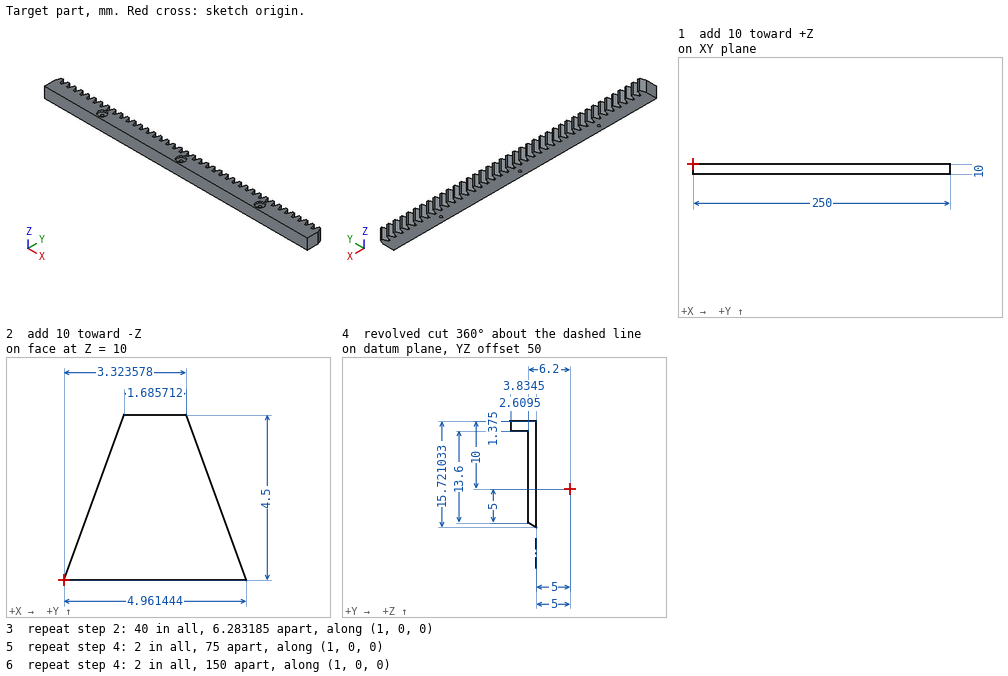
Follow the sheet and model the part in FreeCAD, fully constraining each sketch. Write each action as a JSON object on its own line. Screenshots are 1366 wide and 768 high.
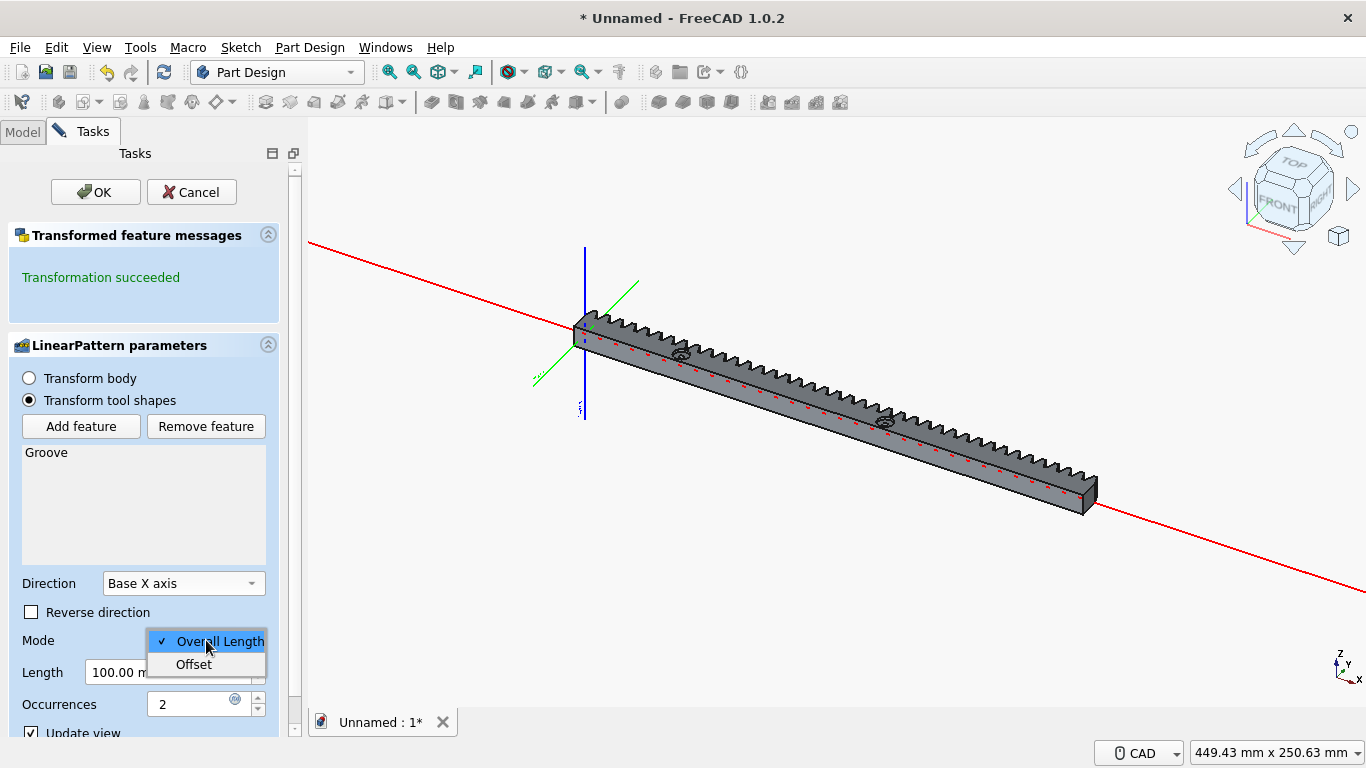
{"action": "left_click", "coordinate": [206, 664]}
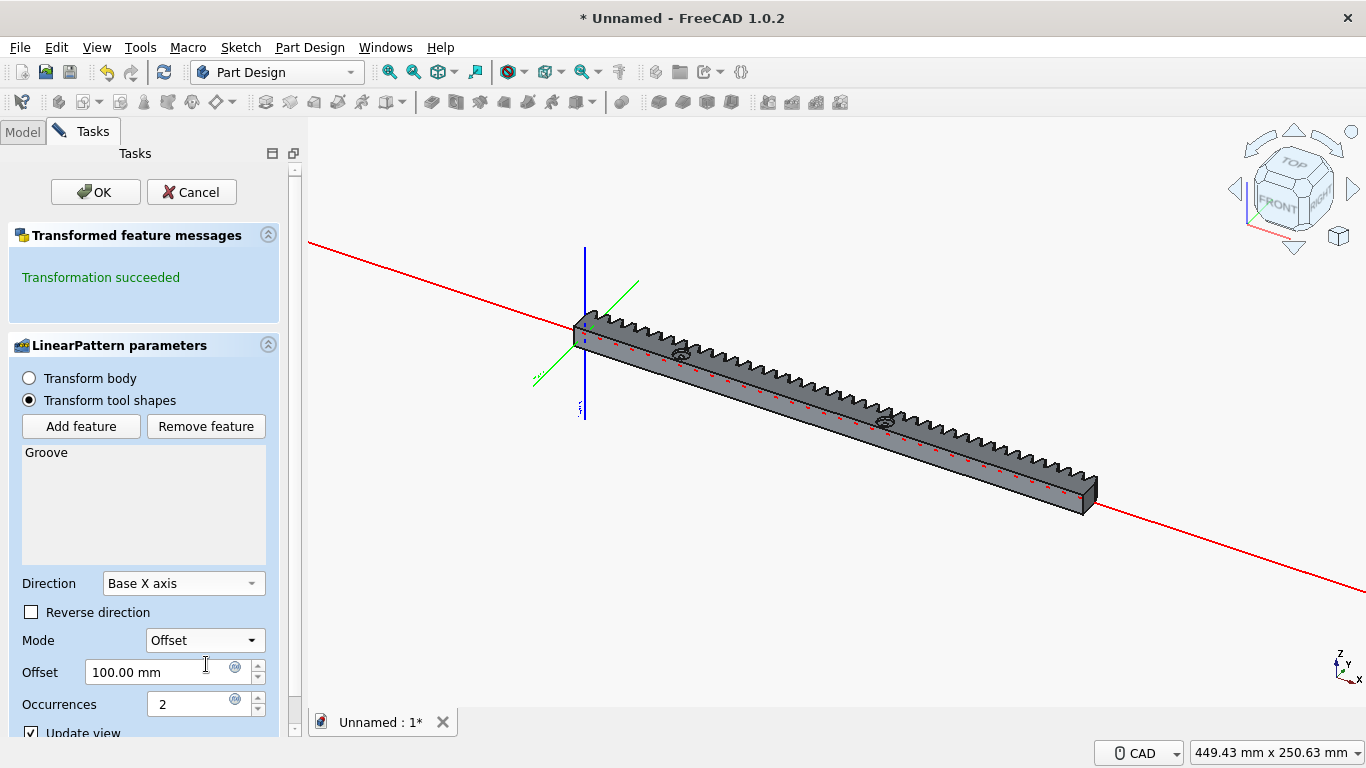
{"action": "triple_click", "coordinate": [168, 672]}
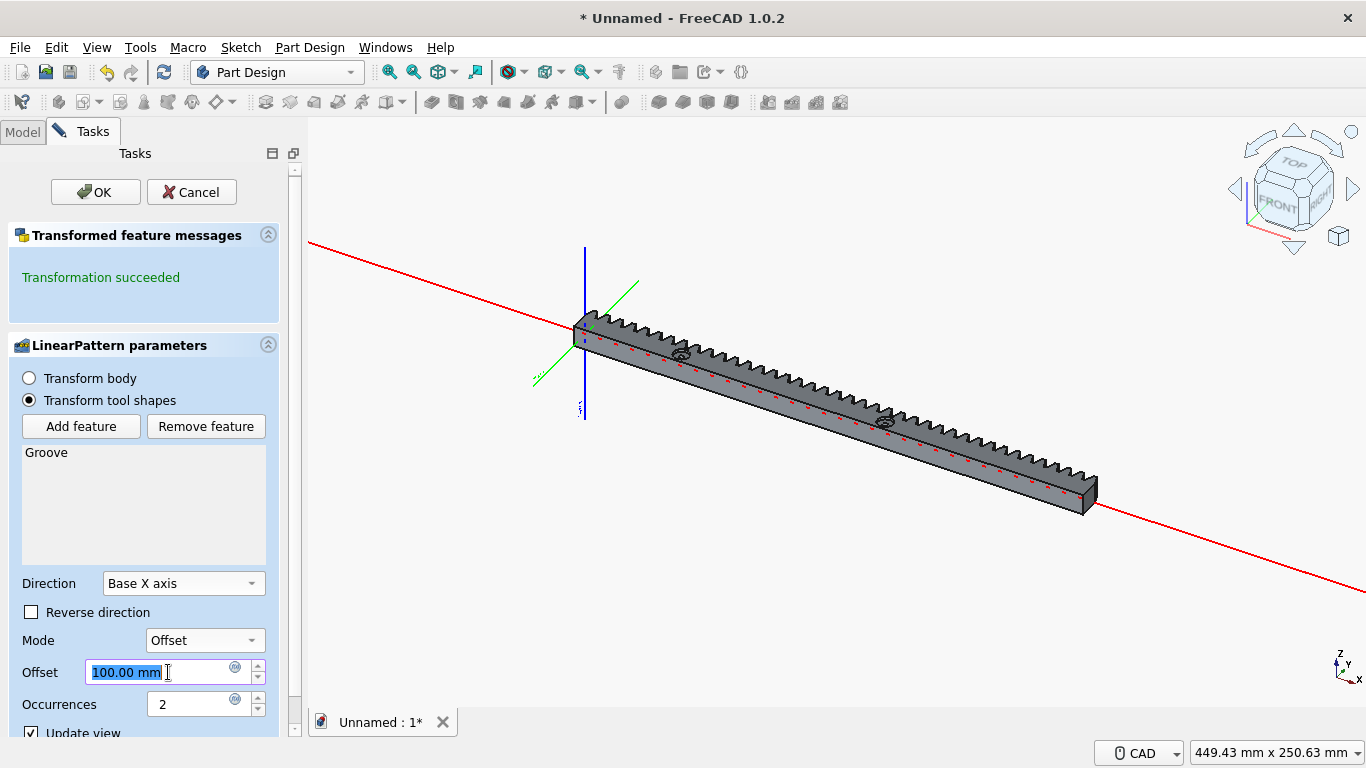
{"action": "type", "text": "75"}
{"action": "key", "text": "Tab"}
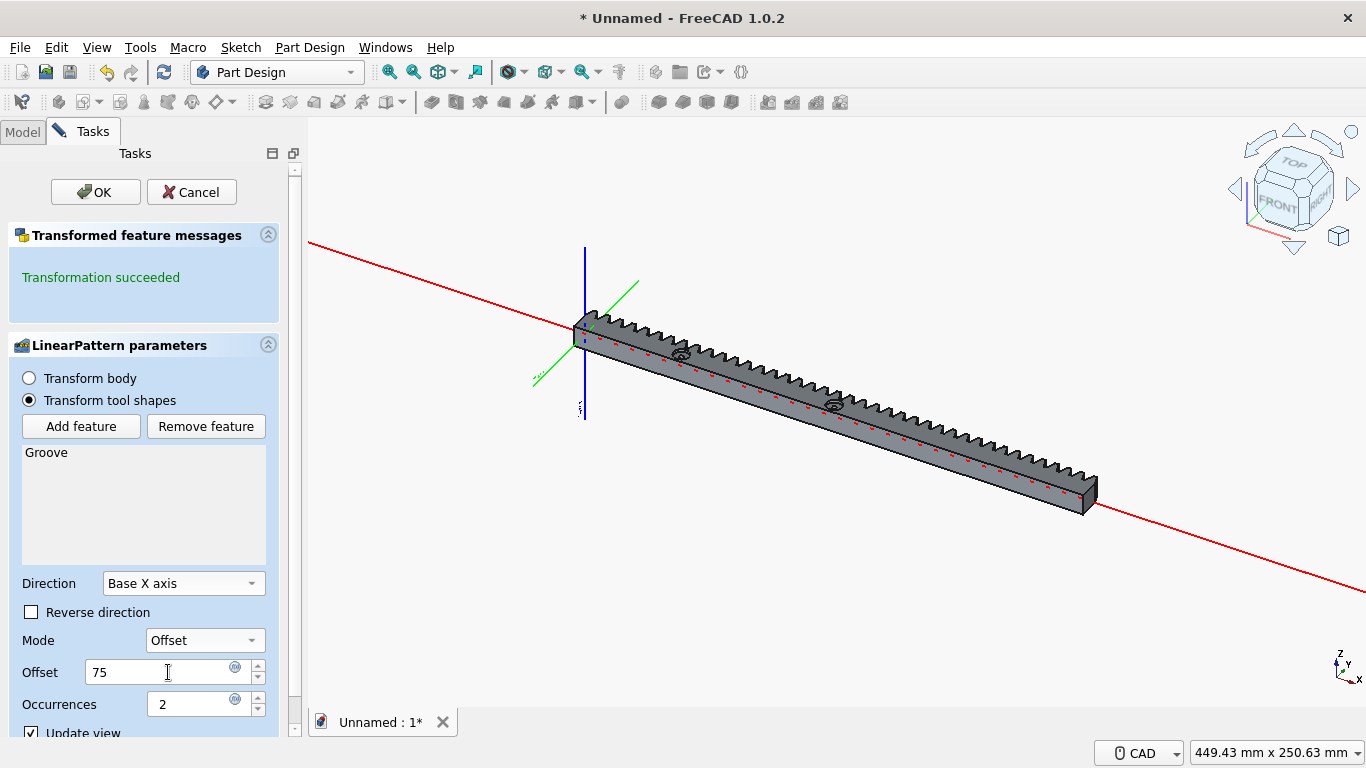
{"action": "triple_click", "coordinate": [198, 704]}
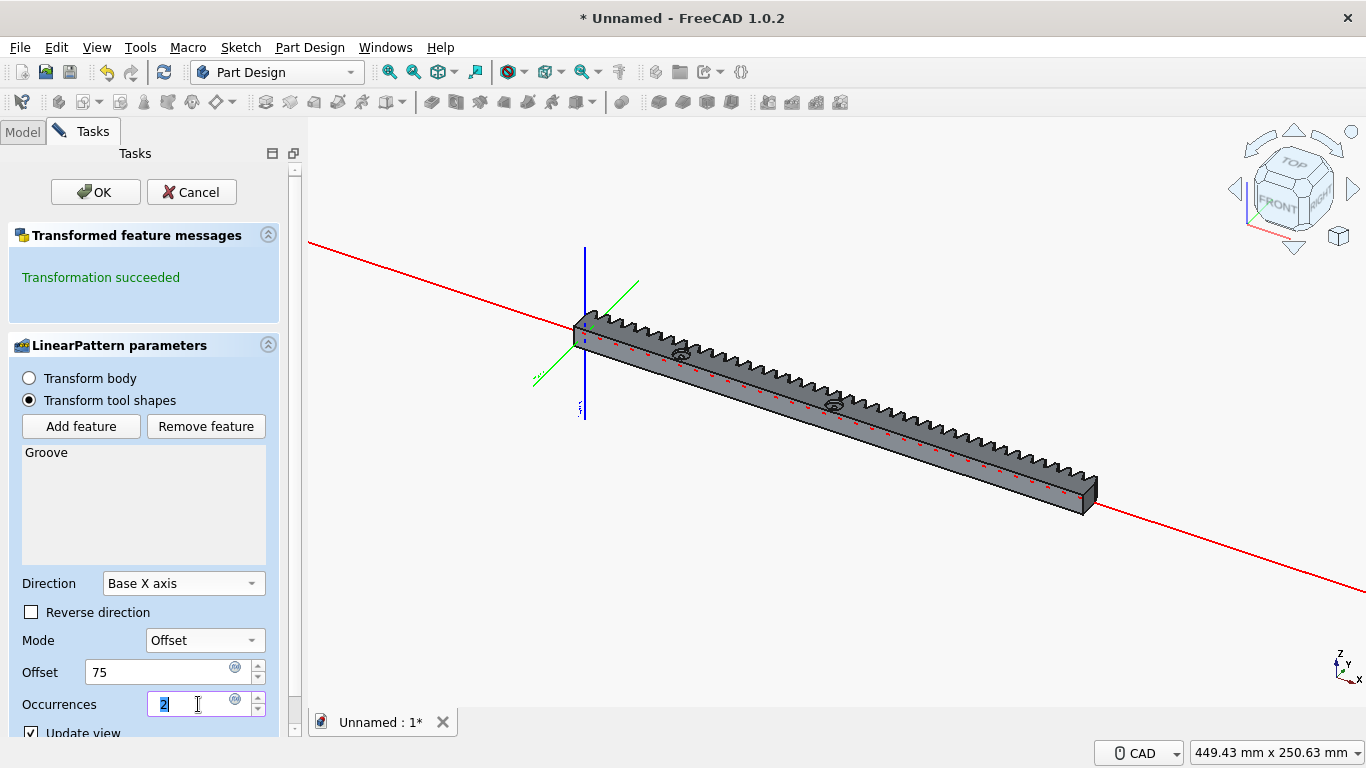
{"action": "type", "text": "2"}
{"action": "key", "text": "Tab"}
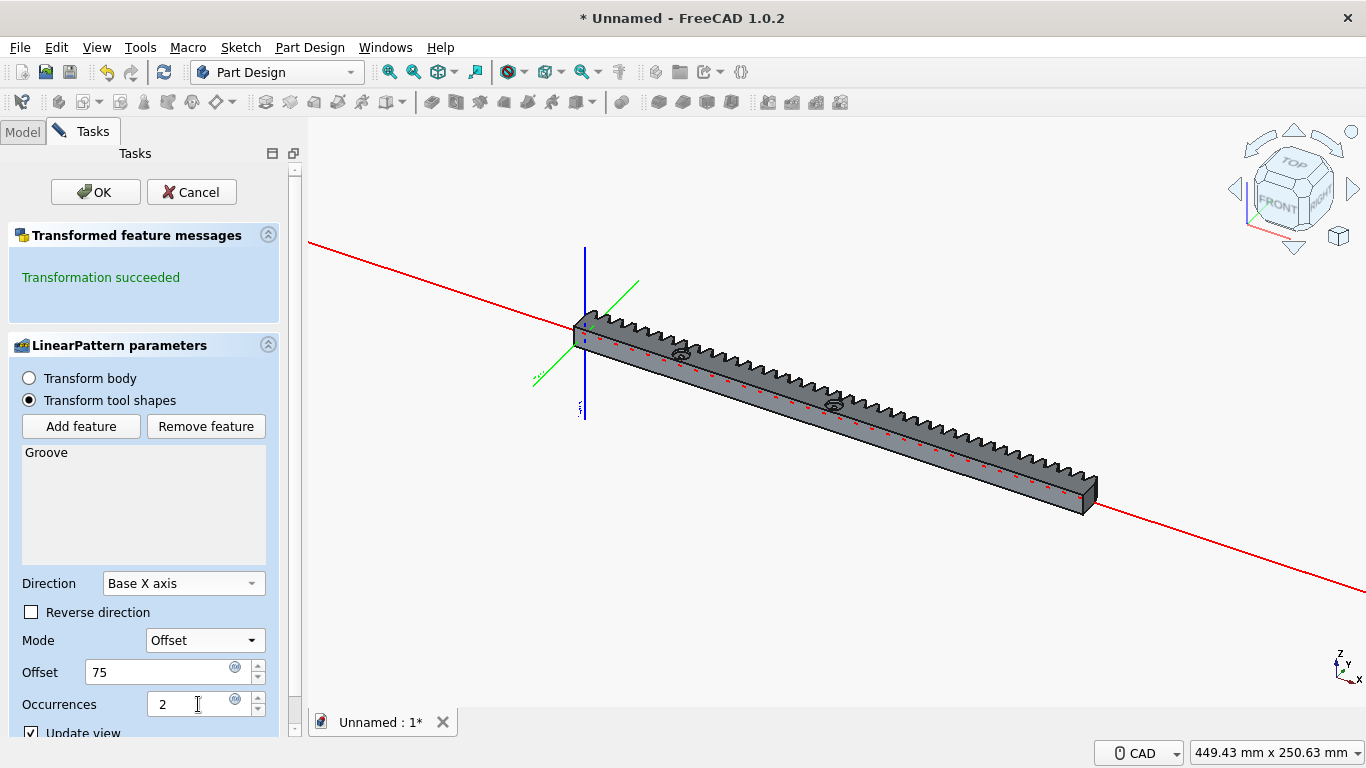
{"action": "left_click", "coordinate": [96, 192]}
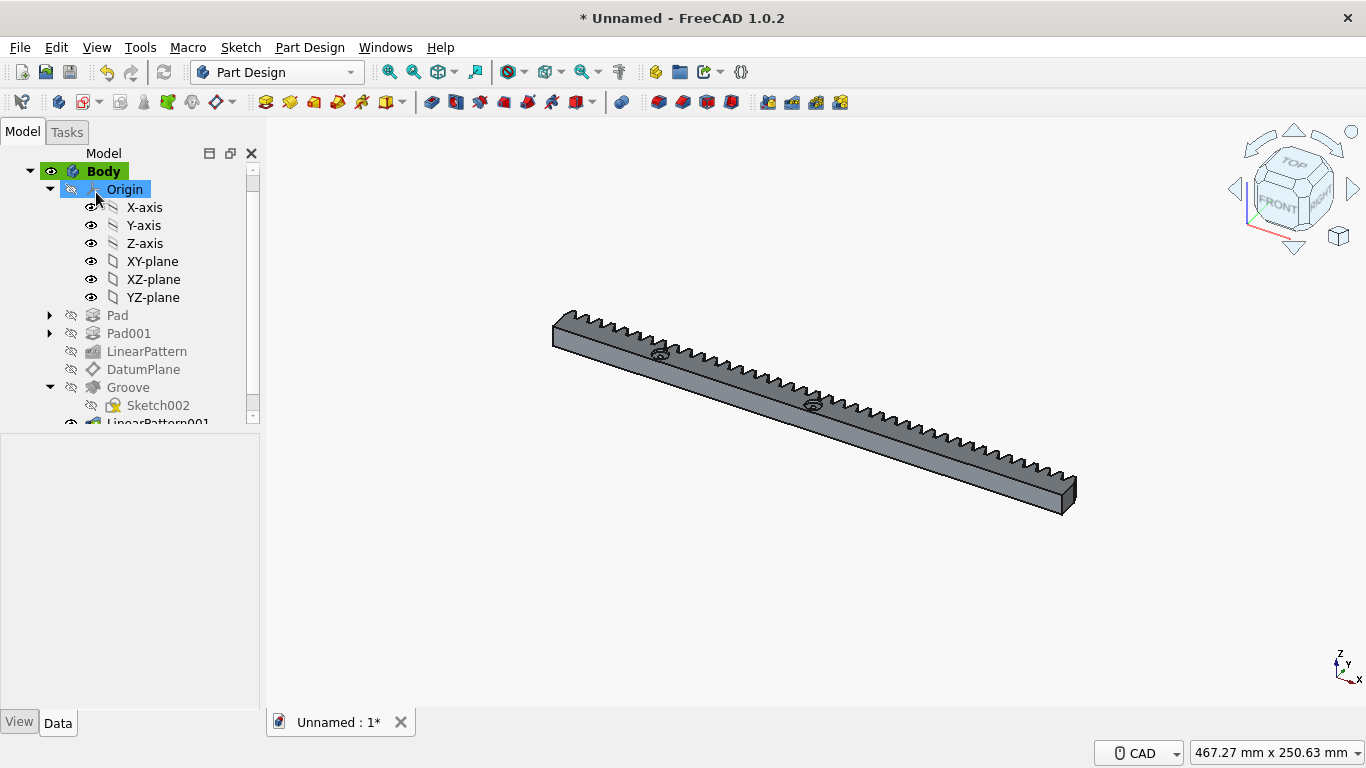
{"action": "left_click", "coordinate": [116, 387]}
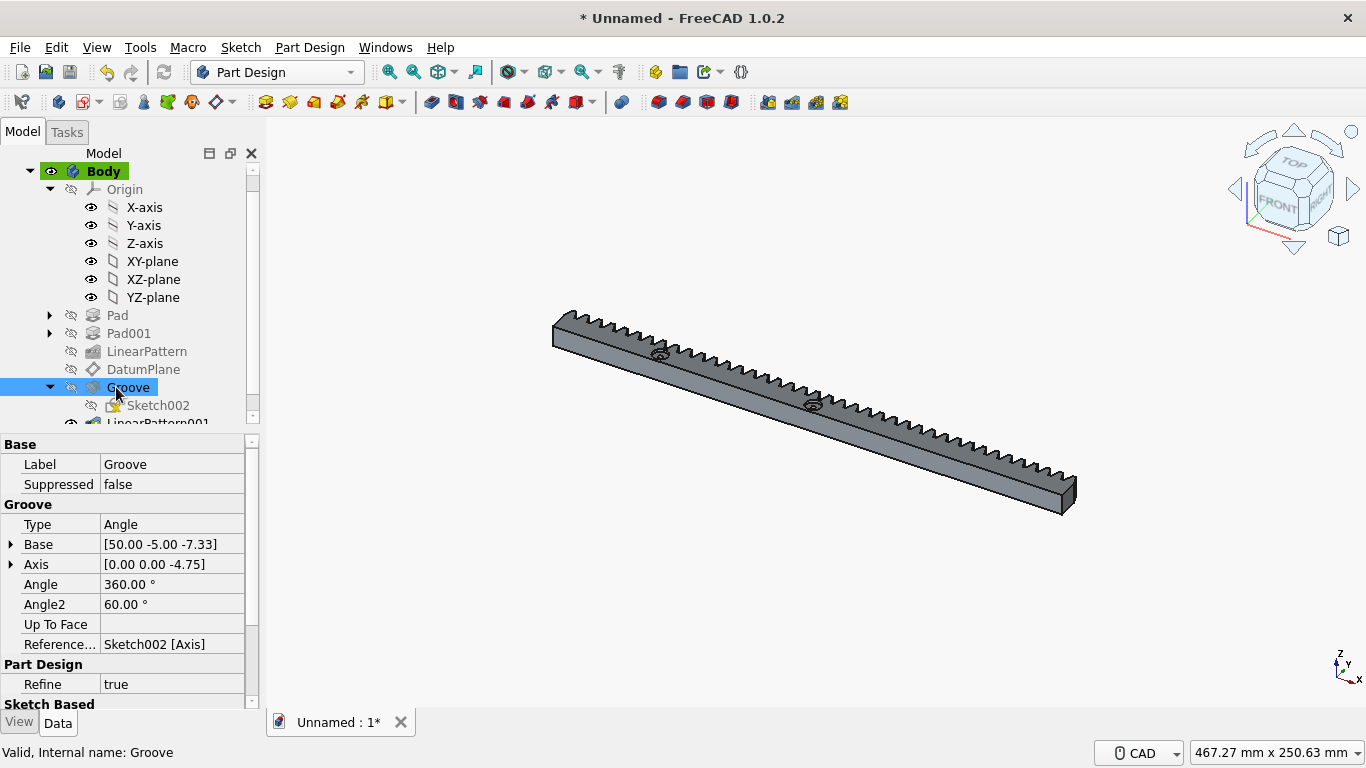
{"action": "left_click", "coordinate": [792, 102]}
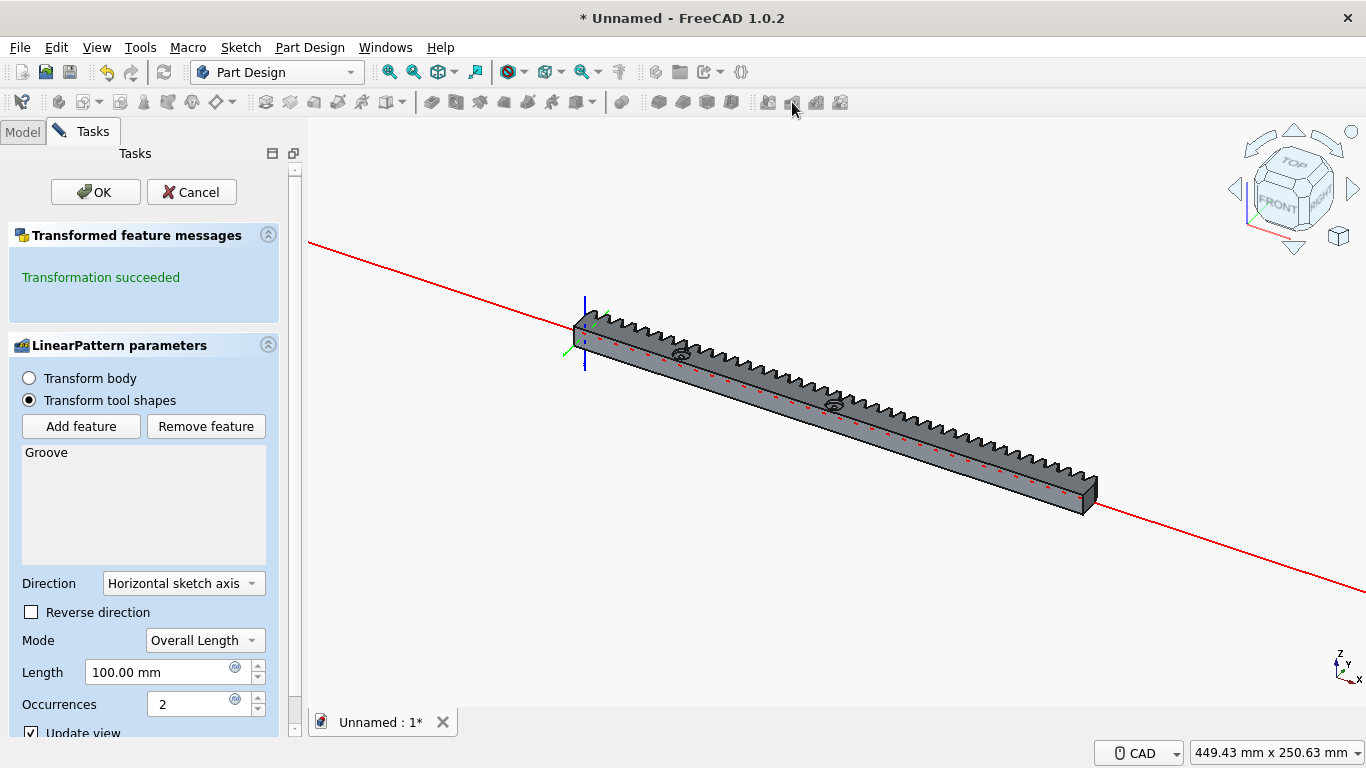
{"action": "left_click", "coordinate": [184, 584]}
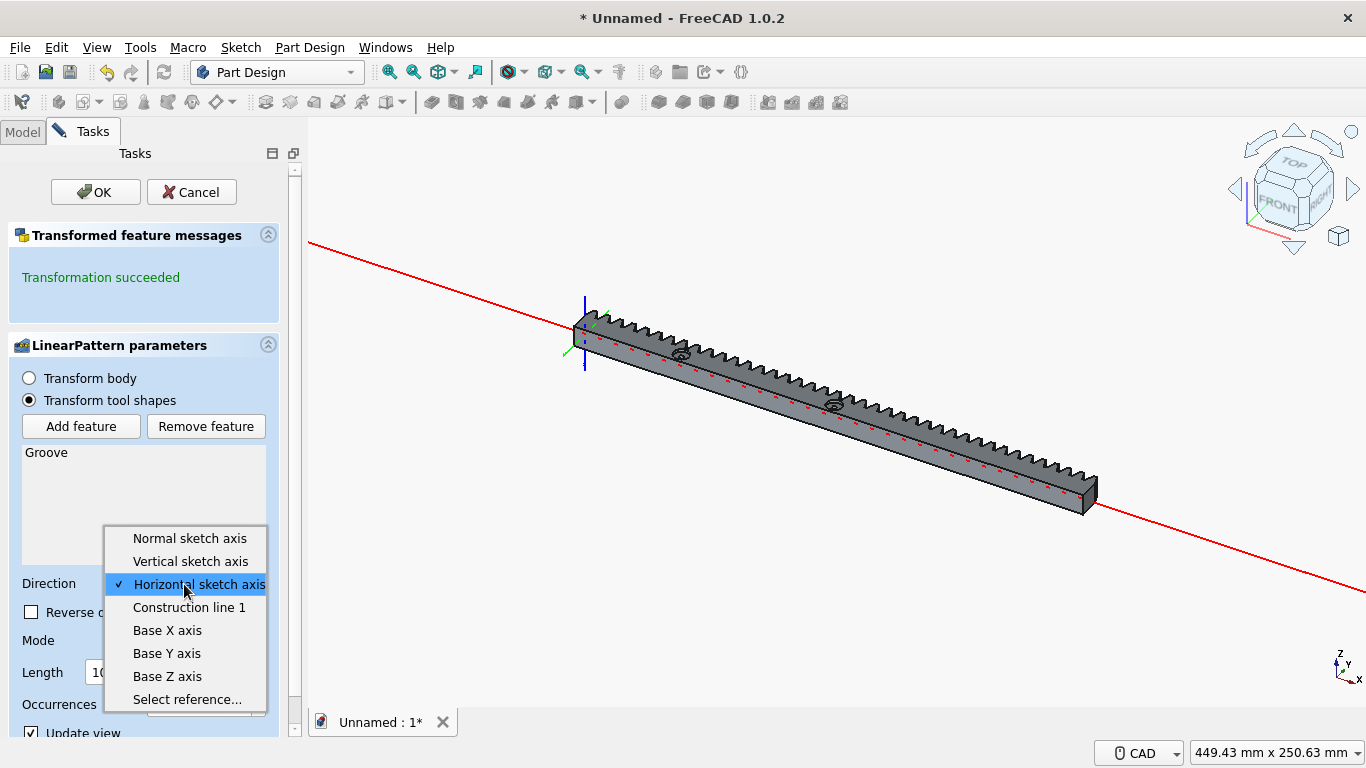
{"action": "left_click", "coordinate": [184, 630]}